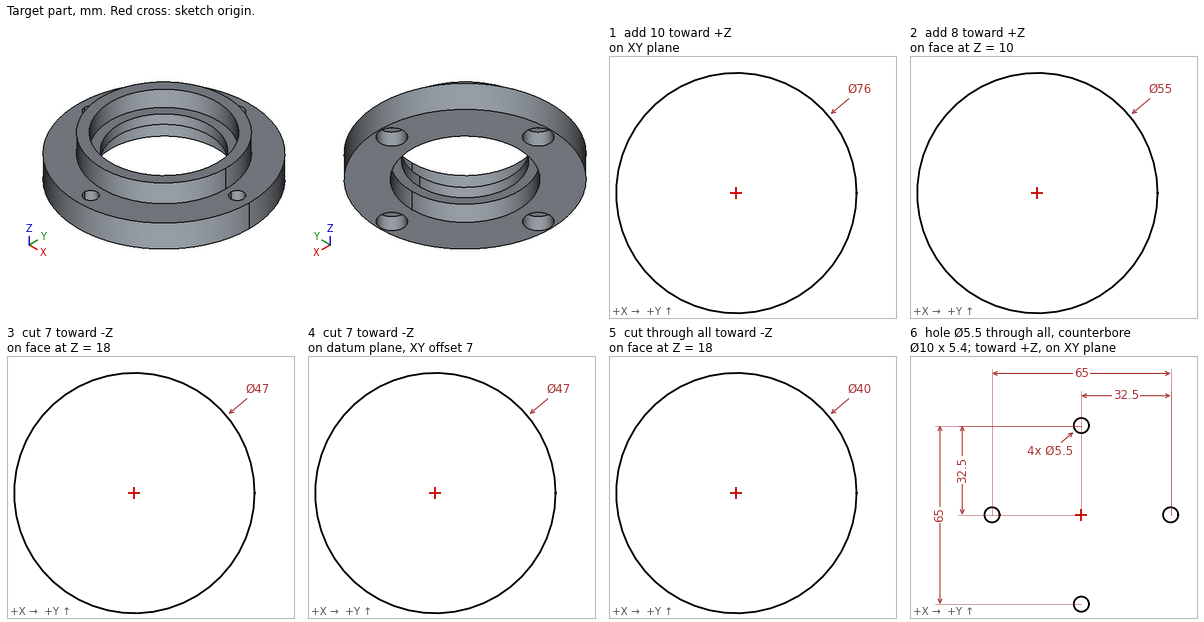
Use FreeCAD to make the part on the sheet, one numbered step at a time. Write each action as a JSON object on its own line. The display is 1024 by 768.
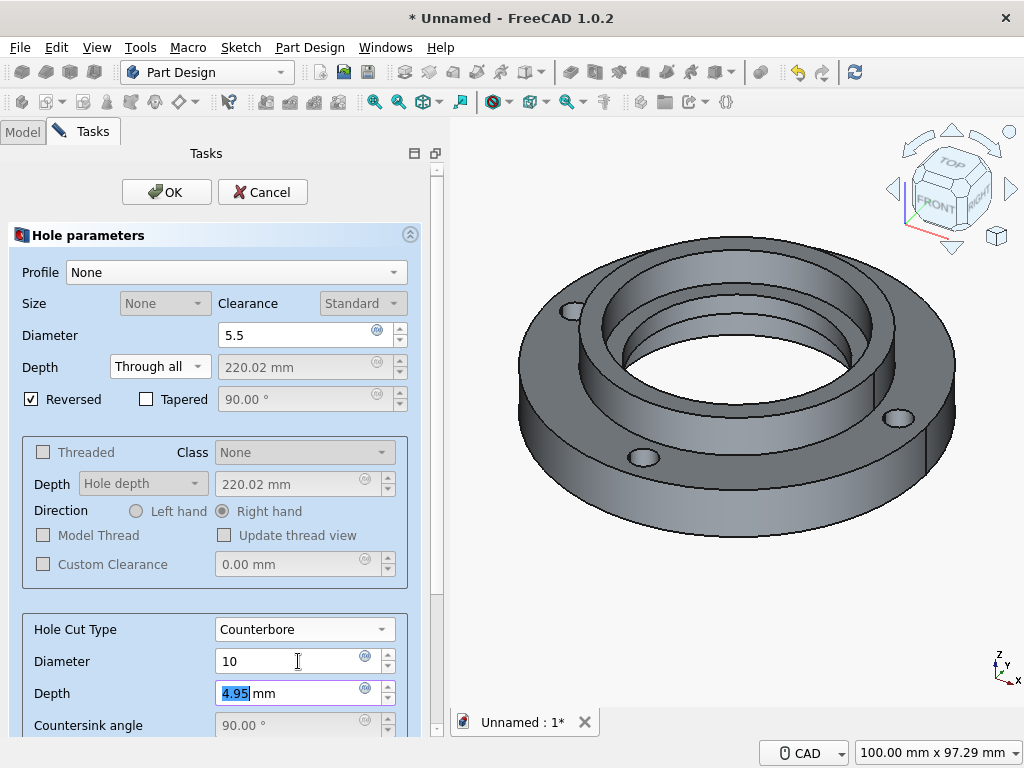
{"action": "type", "text": "5.4"}
{"action": "key", "text": "Tab"}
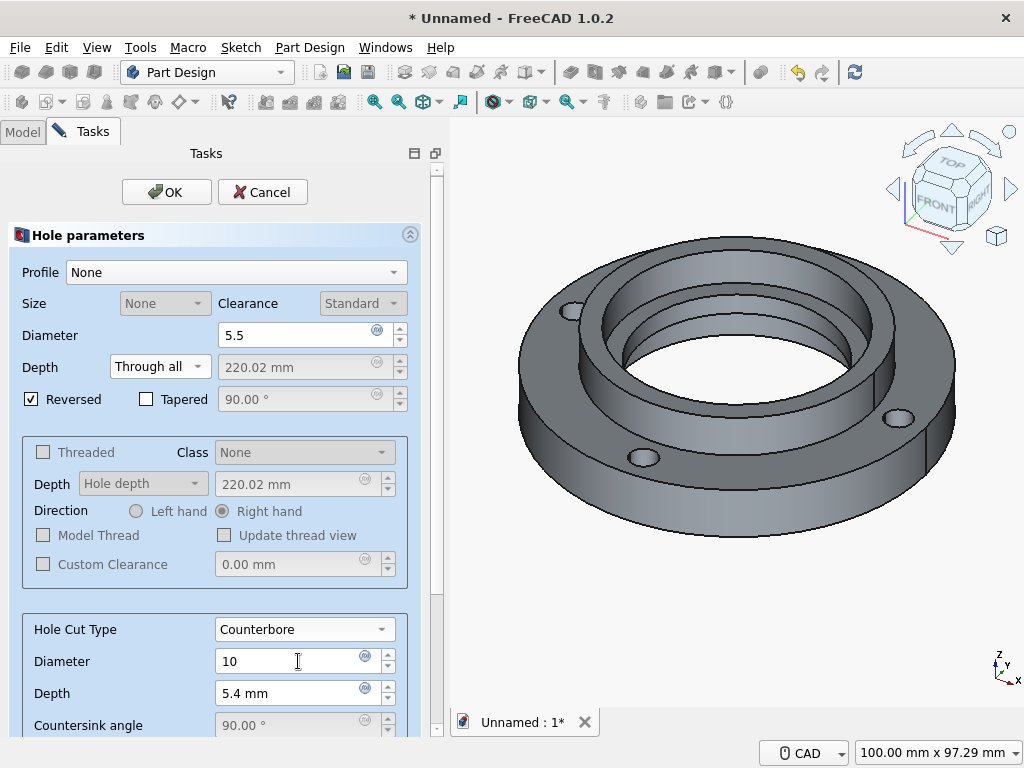
{"action": "left_click", "coordinate": [167, 192]}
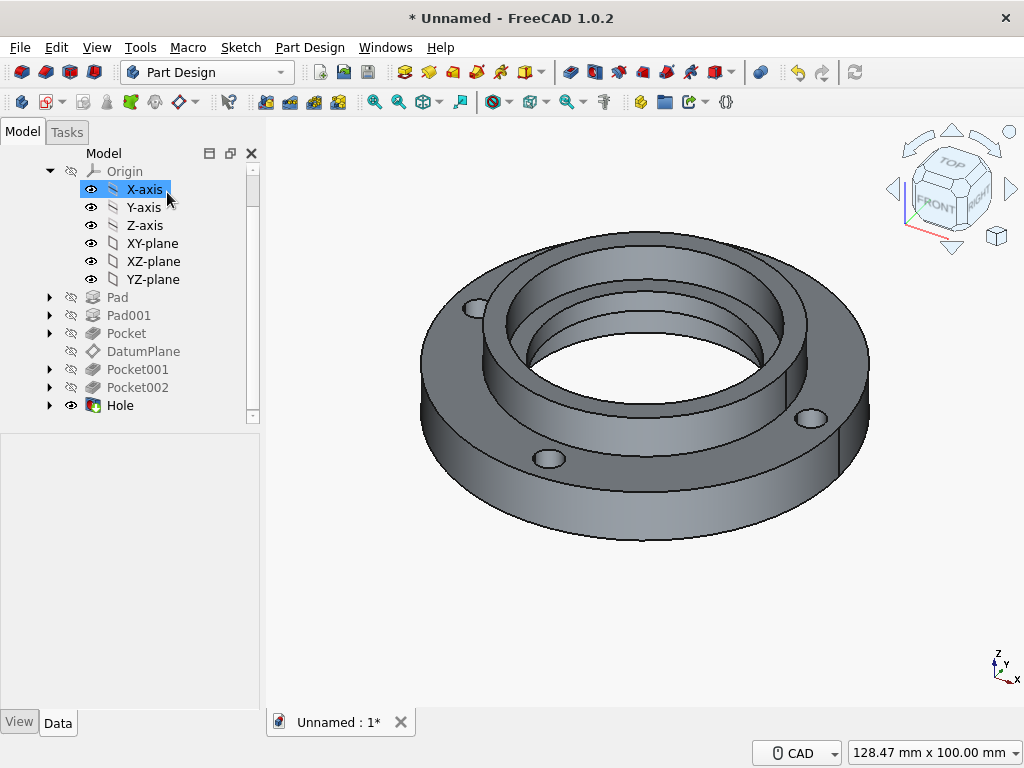
{"action": "key", "text": "0"}